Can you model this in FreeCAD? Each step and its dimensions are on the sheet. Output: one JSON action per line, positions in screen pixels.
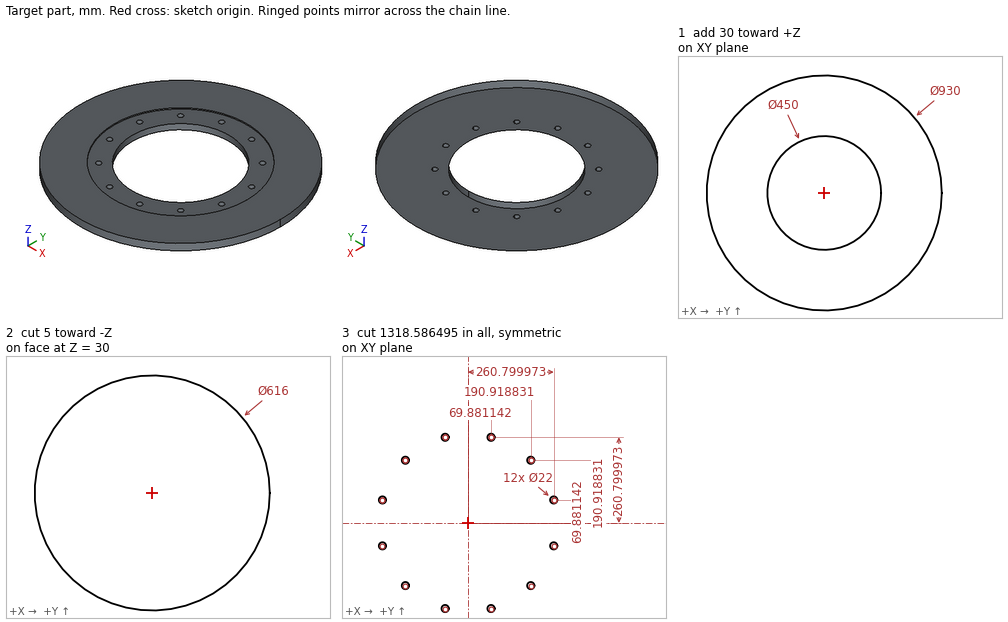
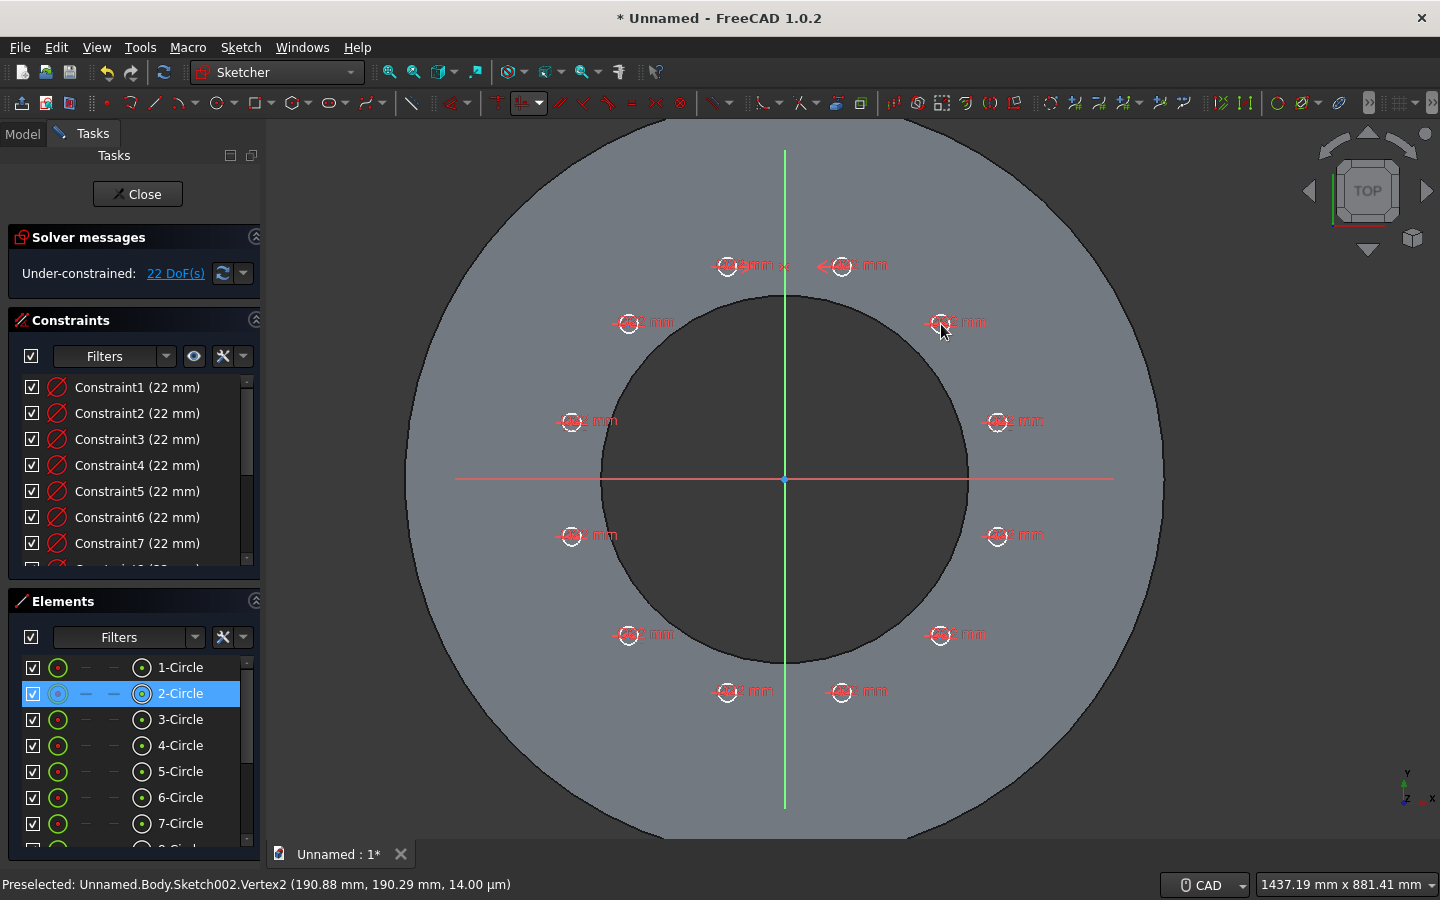
{"action": "left_click", "coordinate": [629, 324]}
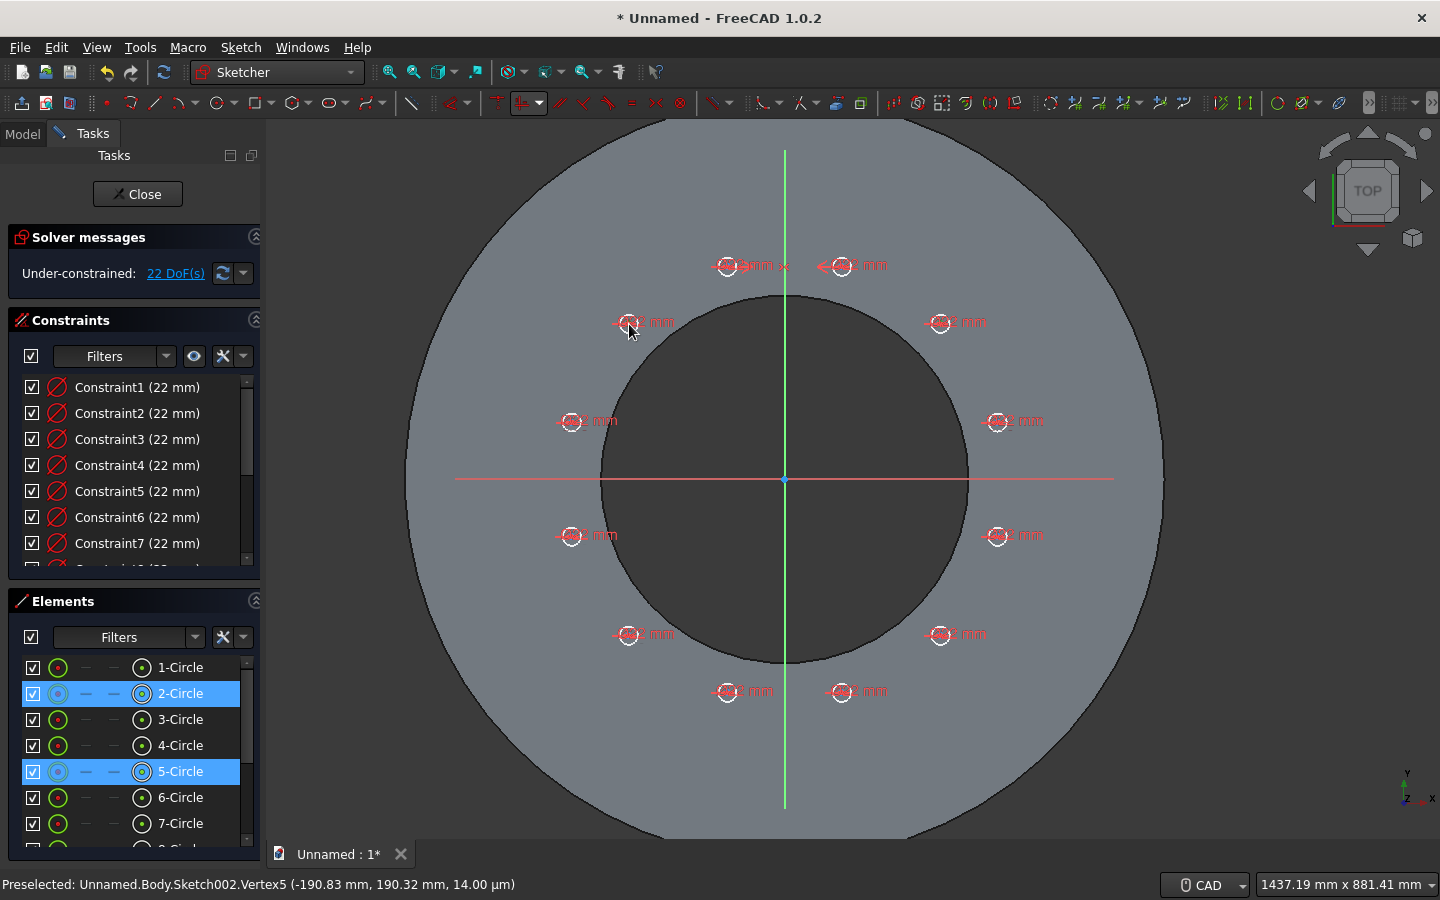
{"action": "left_click", "coordinate": [785, 764]}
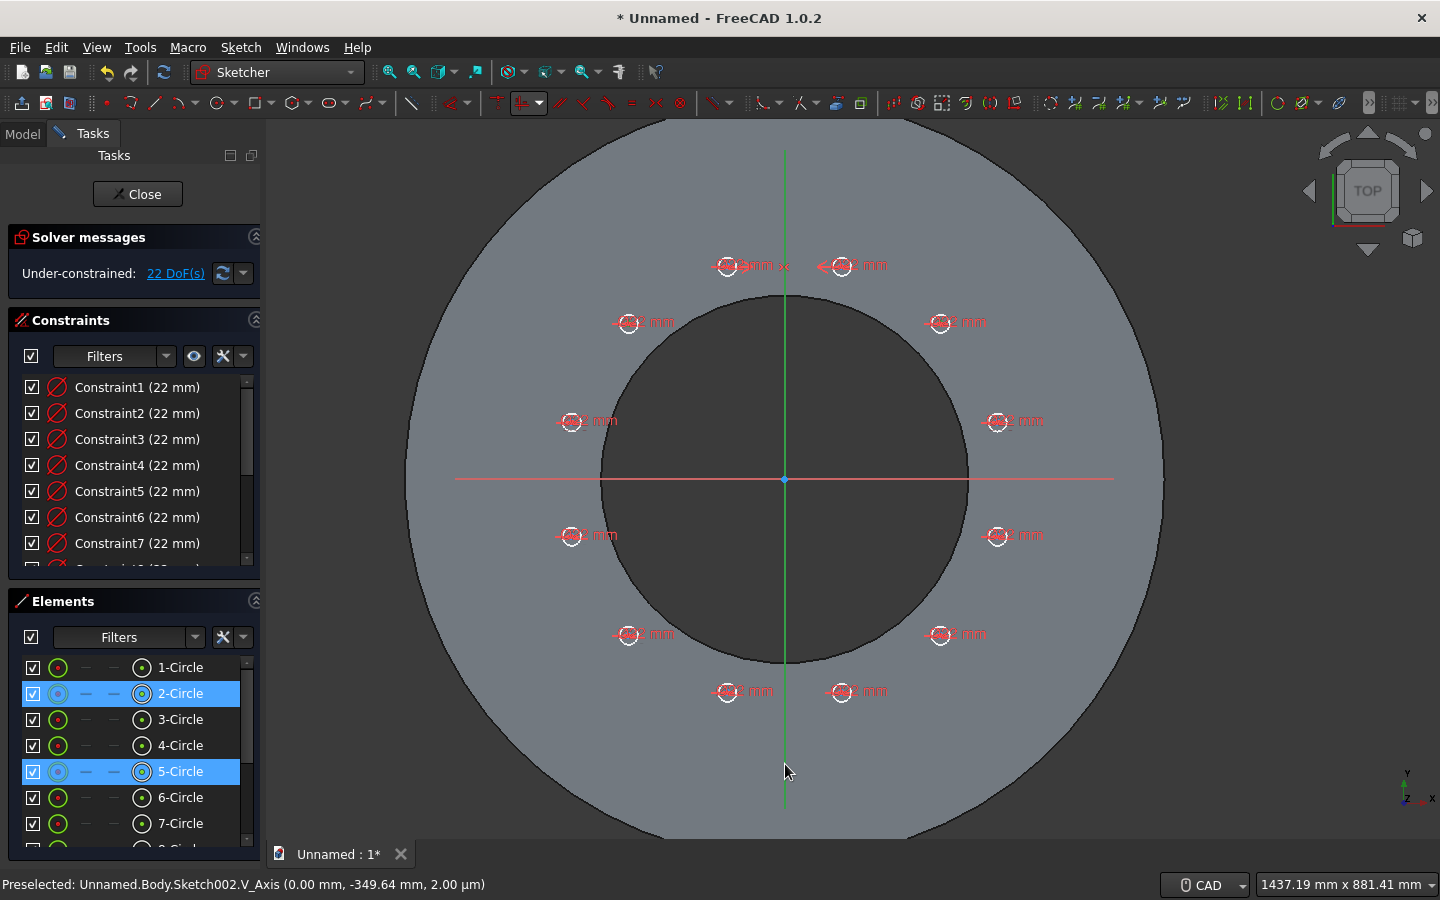
{"action": "left_click", "coordinate": [656, 104]}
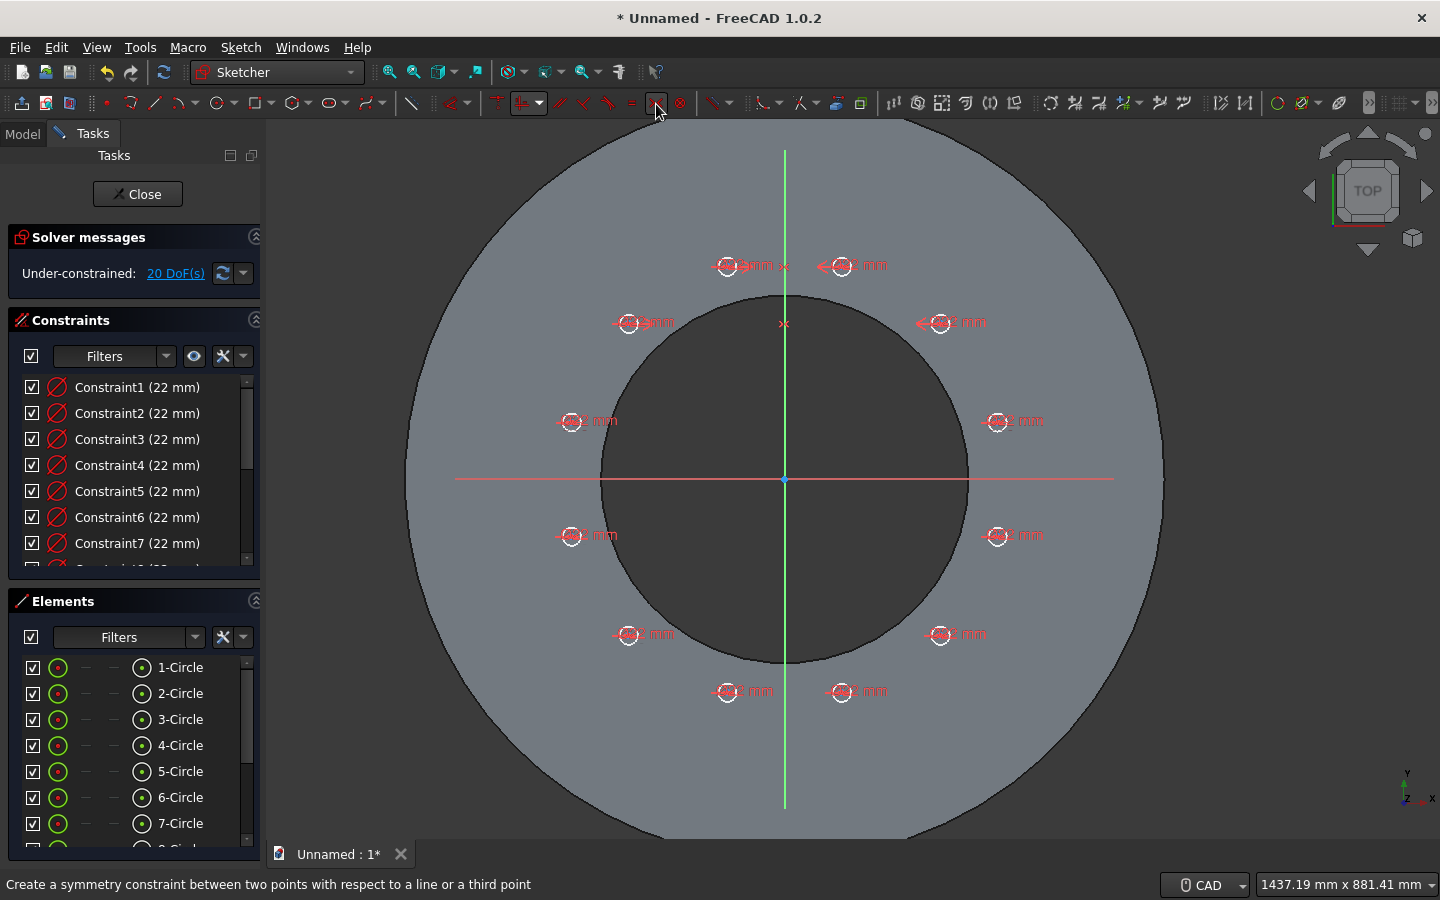
{"action": "left_click", "coordinate": [998, 423]}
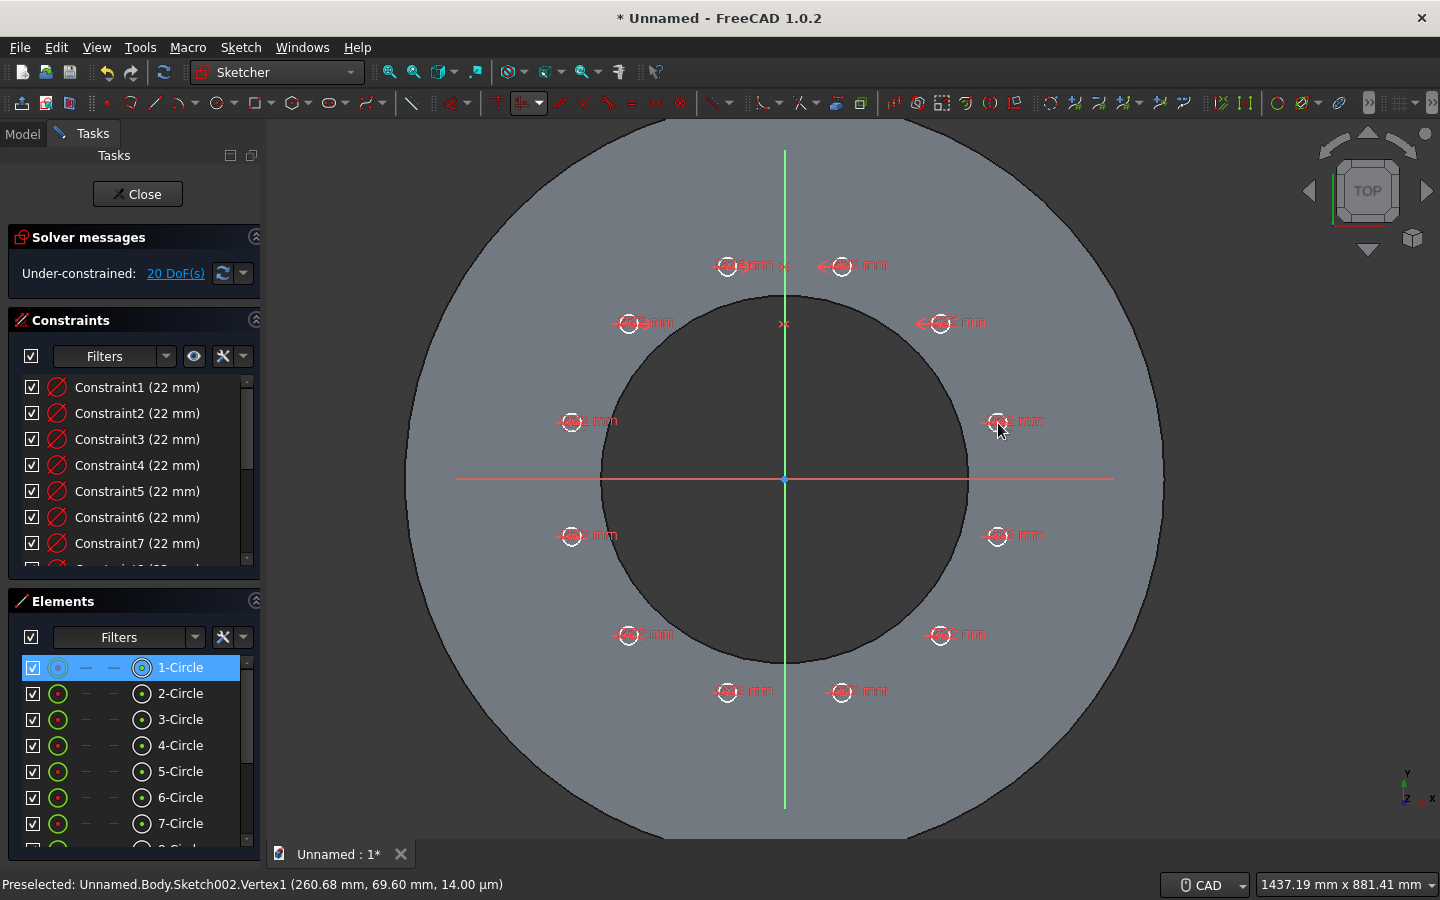
{"action": "left_click", "coordinate": [572, 423]}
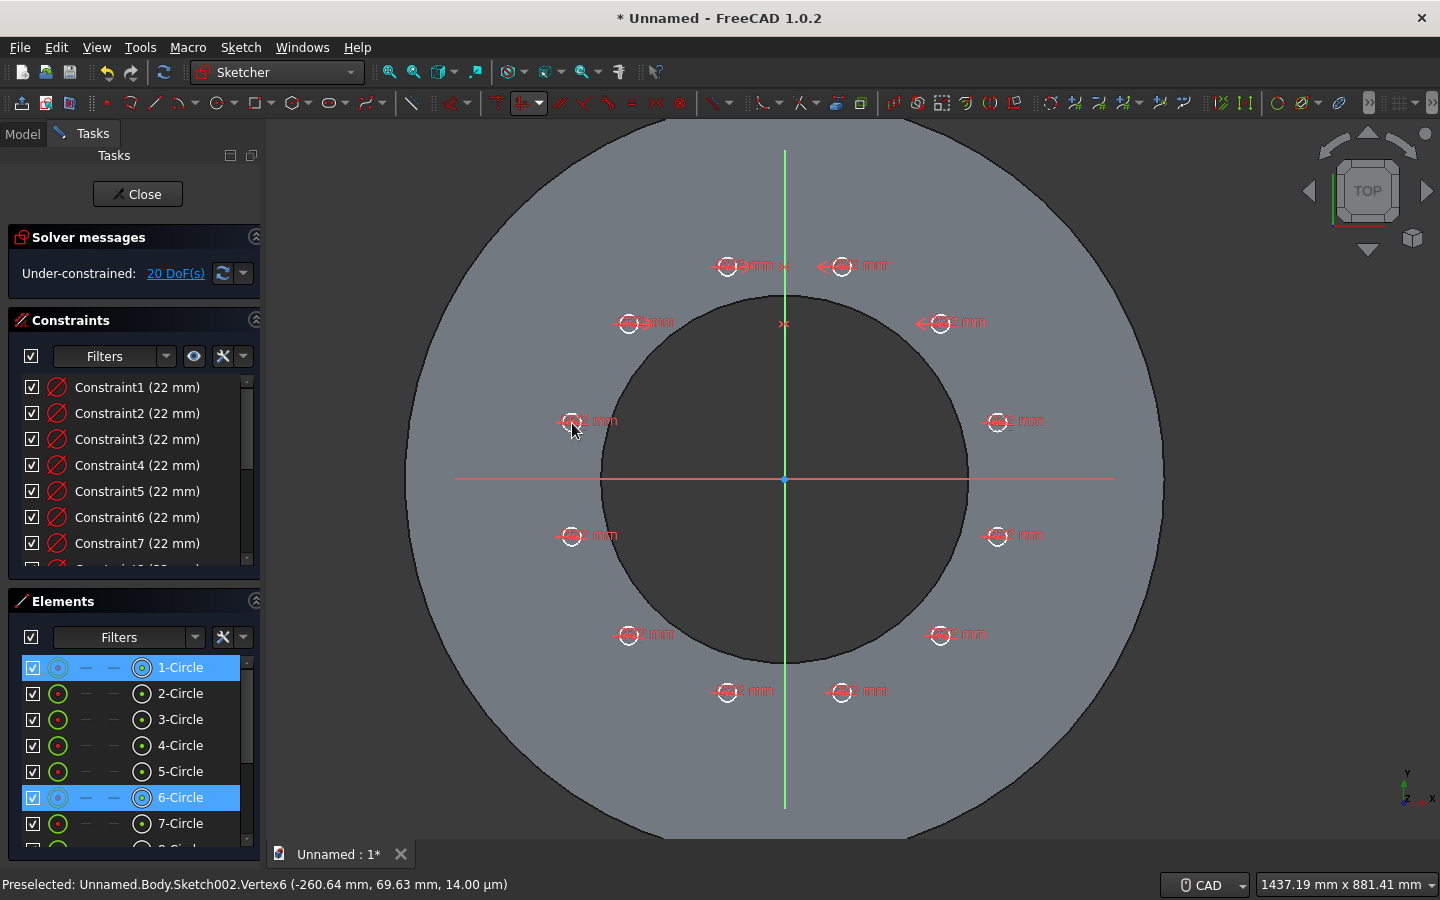
{"action": "left_click", "coordinate": [785, 764]}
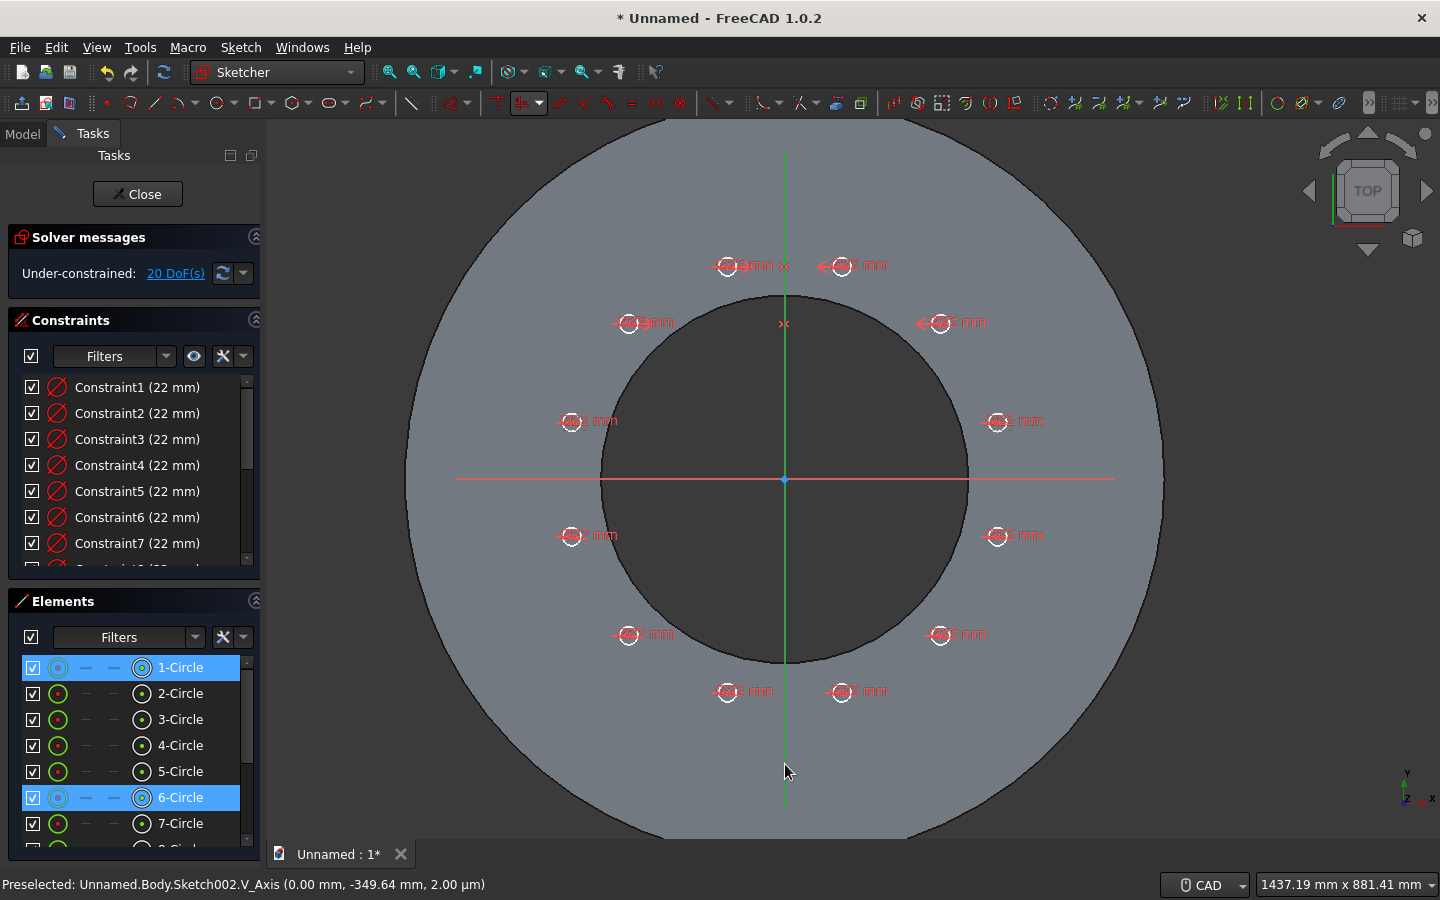
{"action": "left_click", "coordinate": [656, 104]}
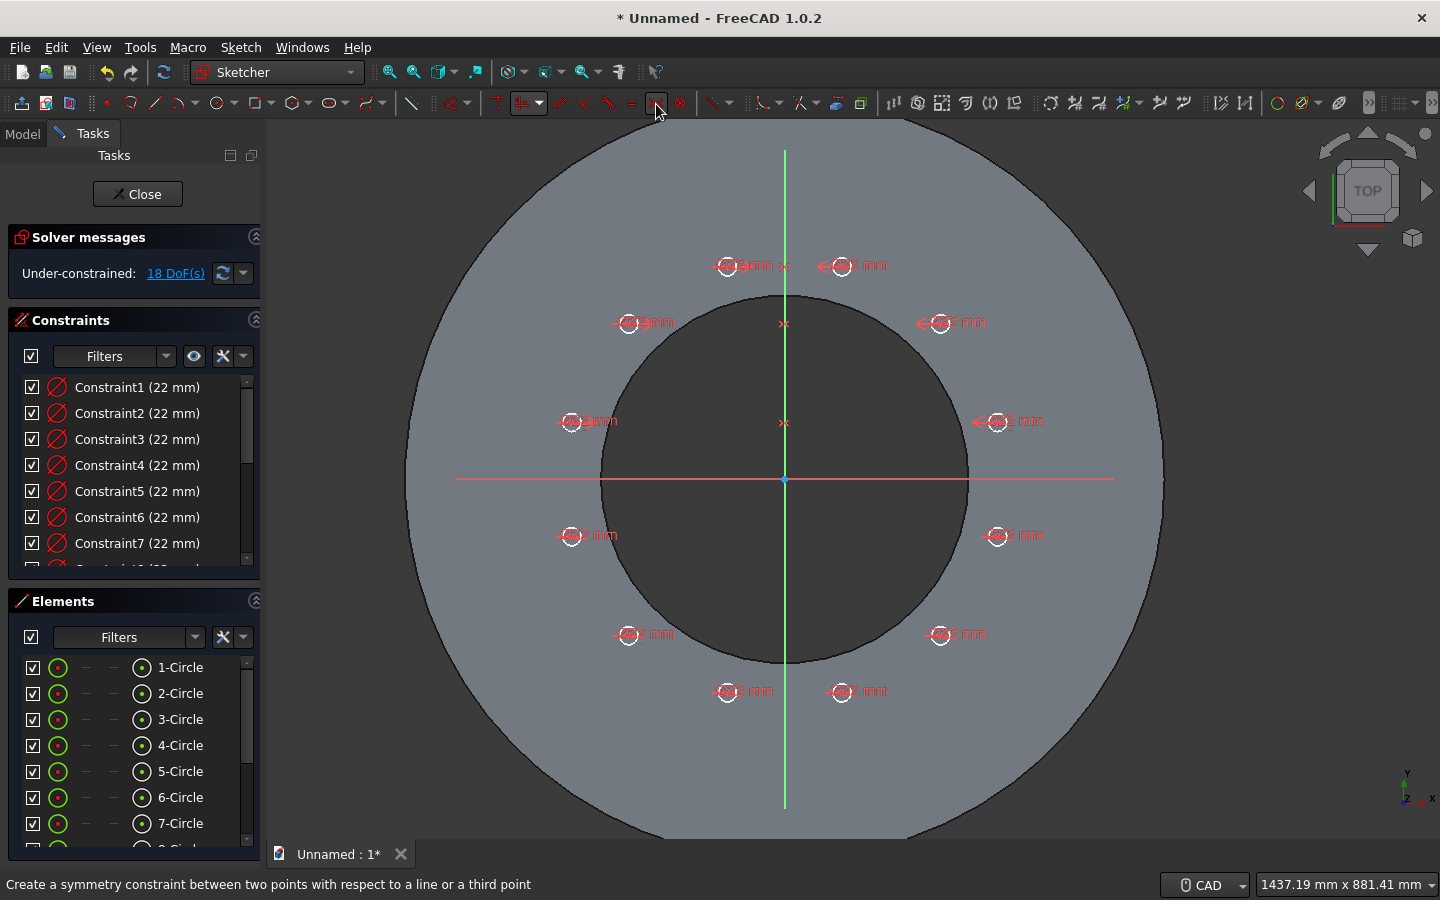
{"action": "left_click", "coordinate": [572, 423]}